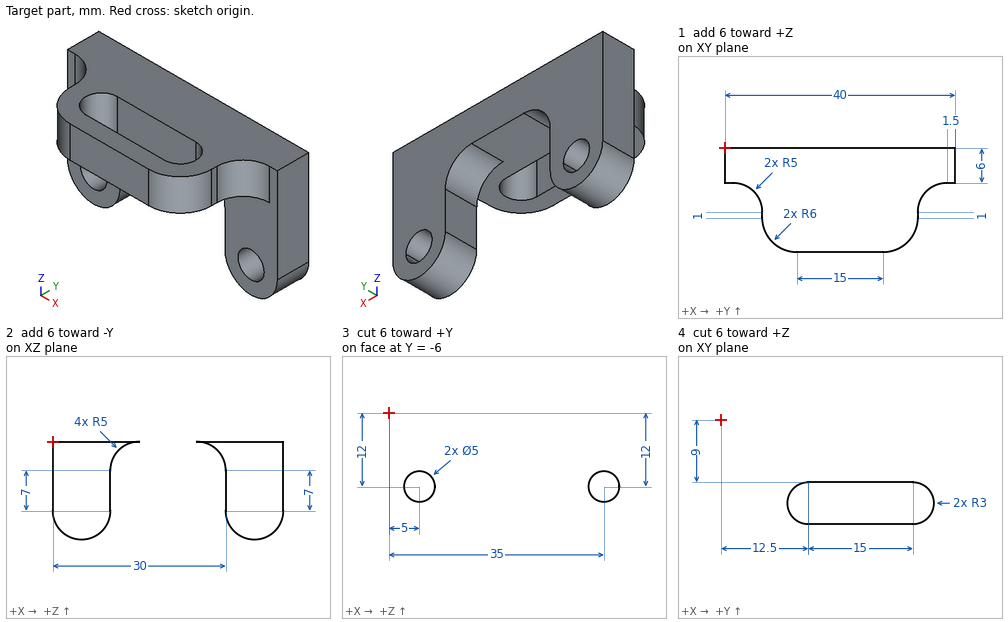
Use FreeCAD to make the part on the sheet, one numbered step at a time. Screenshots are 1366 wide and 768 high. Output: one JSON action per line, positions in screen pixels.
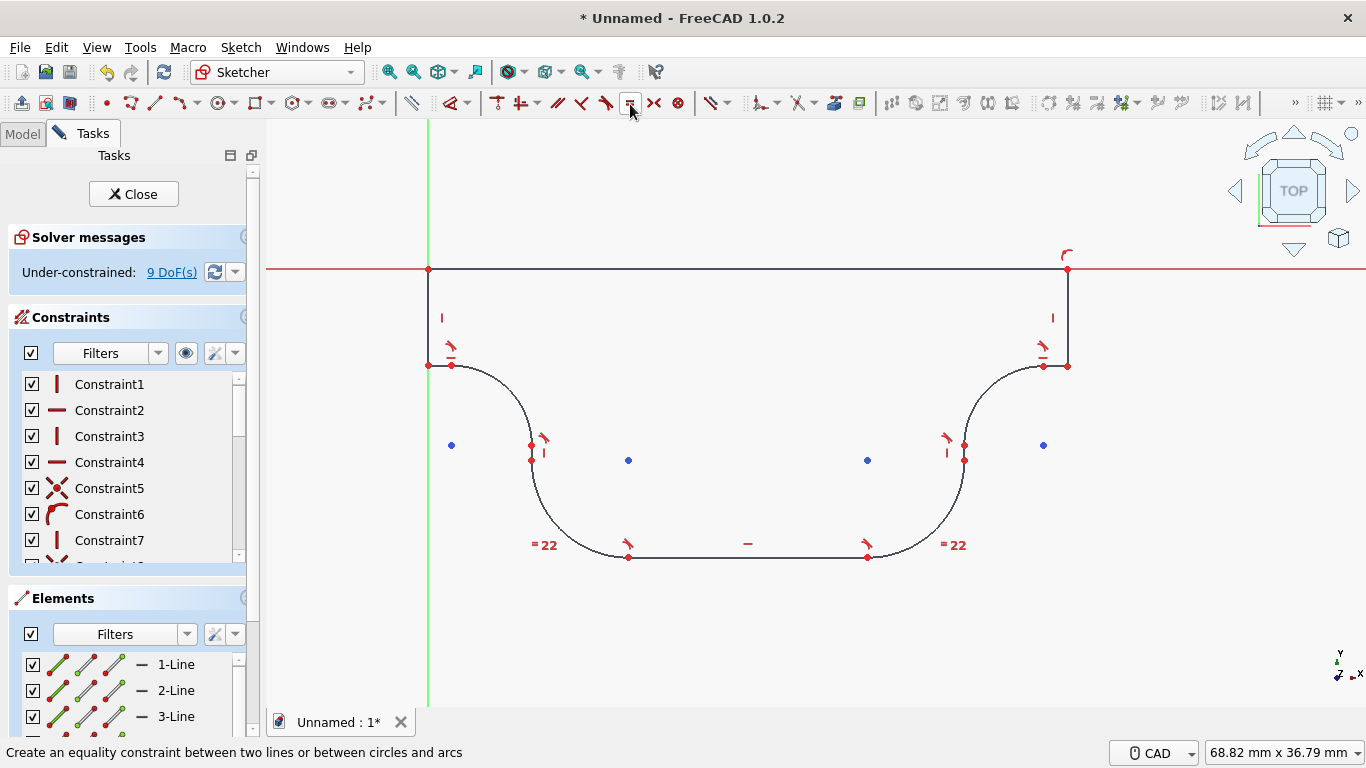
{"action": "left_click", "coordinate": [1008, 375]}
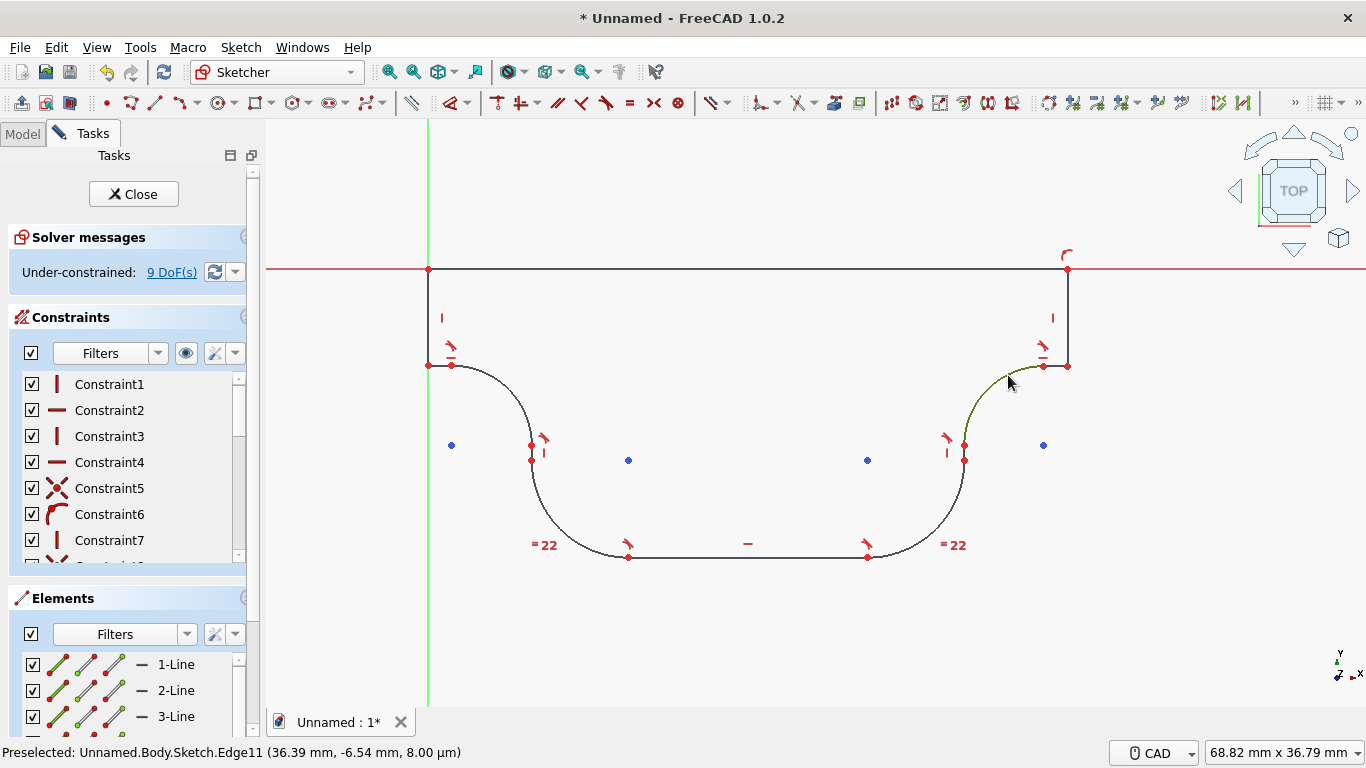
{"action": "left_click", "coordinate": [523, 409]}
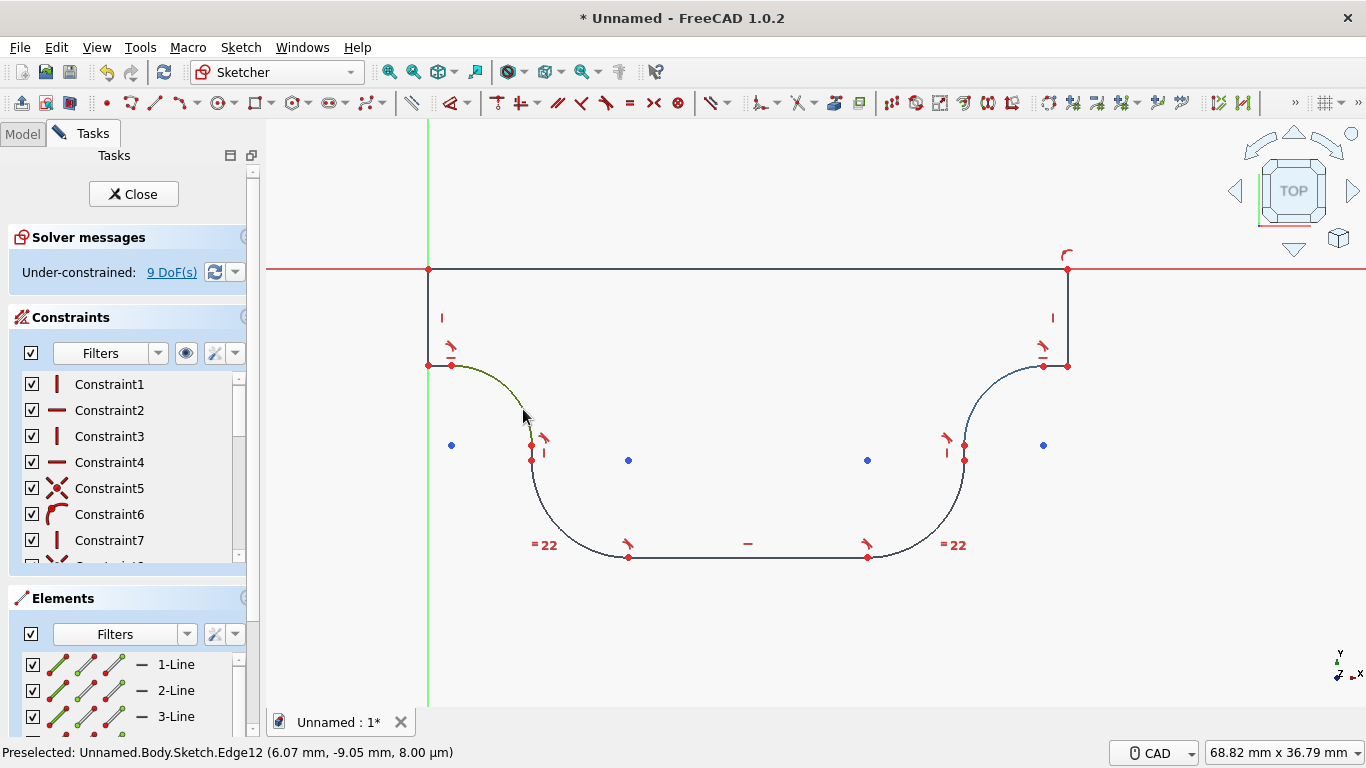
{"action": "key", "text": "e"}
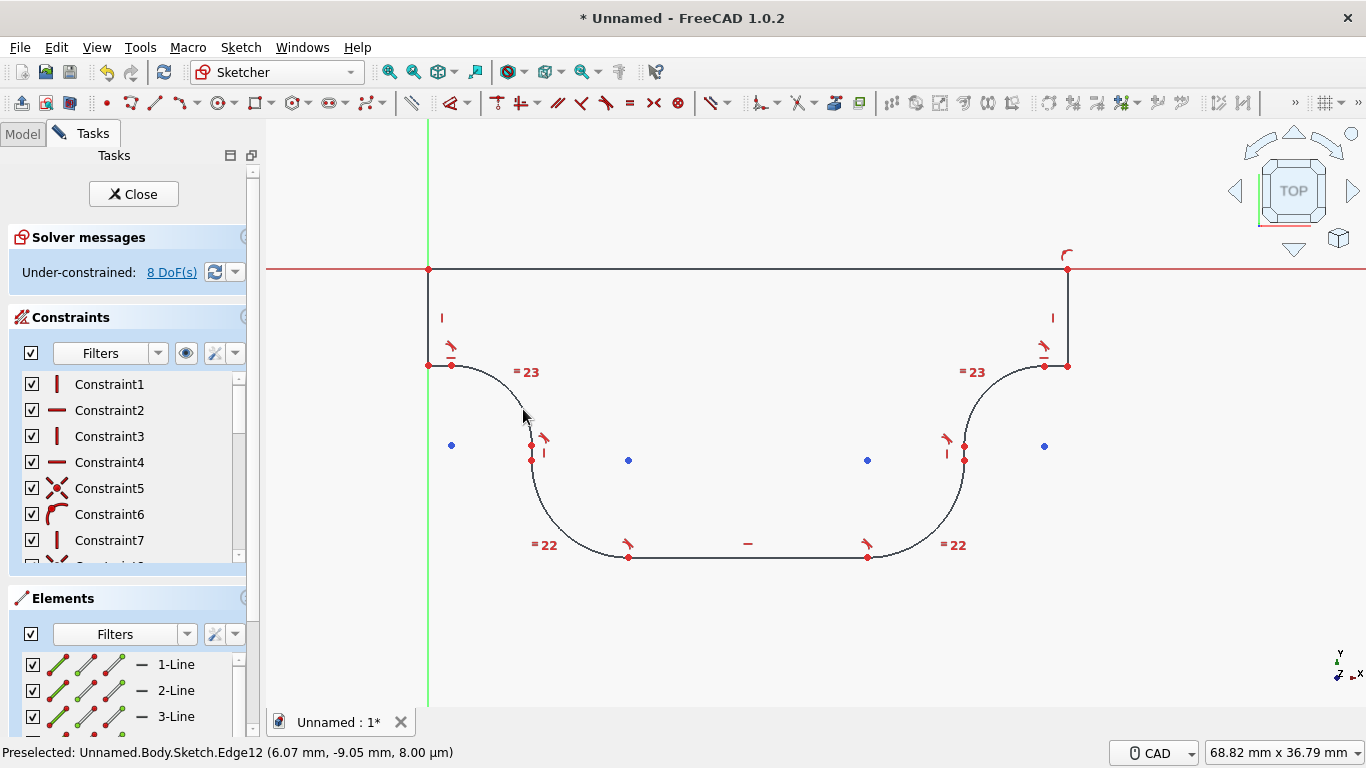
{"action": "key", "text": "d"}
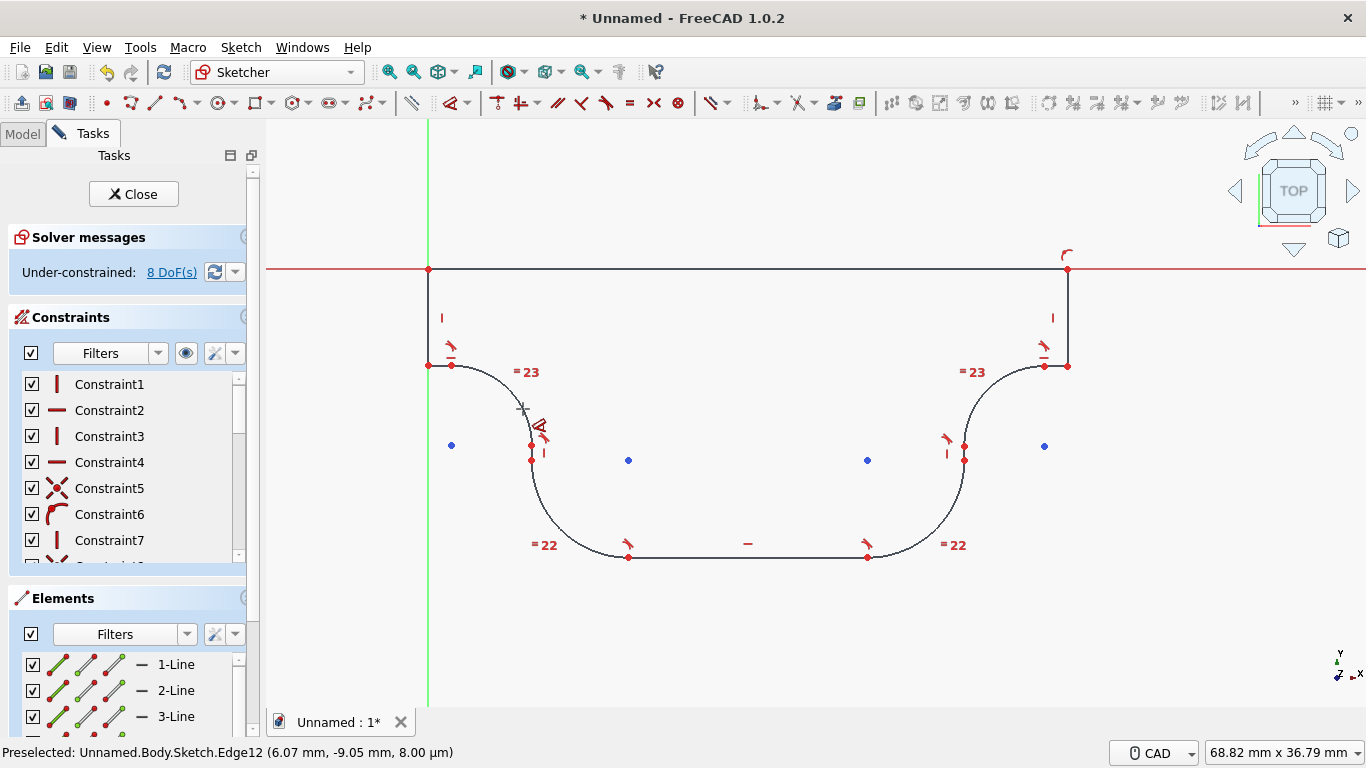
{"action": "left_click", "coordinate": [542, 505]}
{"action": "left_click", "coordinate": [513, 520]}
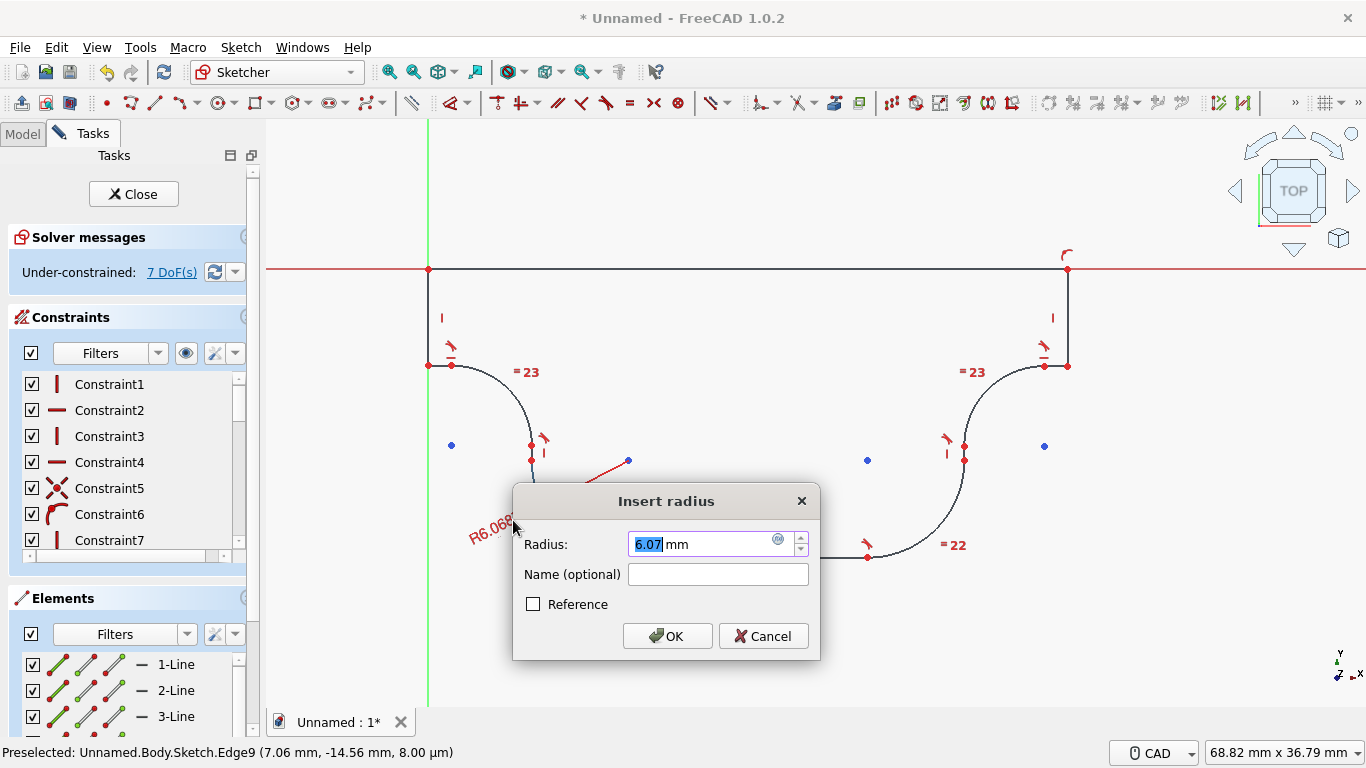
{"action": "type", "text": "6"}
{"action": "key", "text": "Return"}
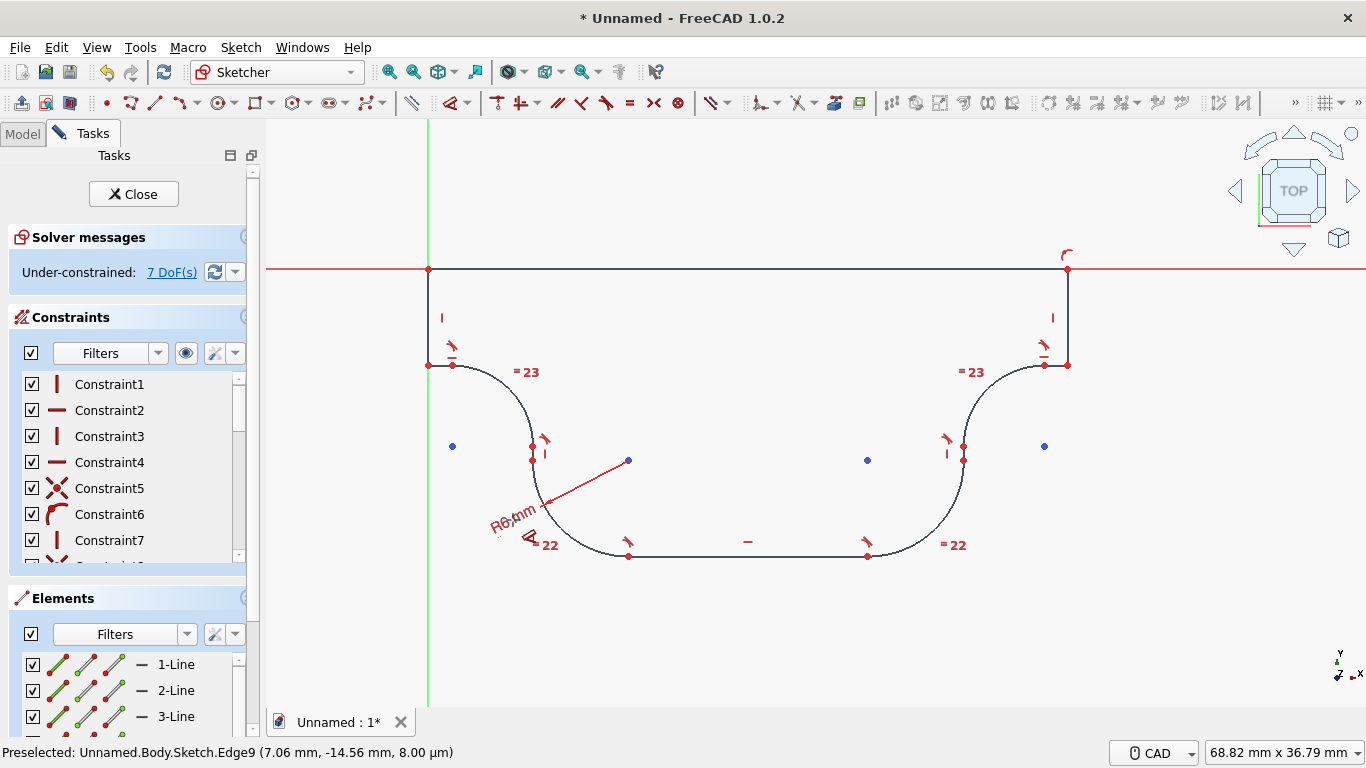
{"action": "left_click", "coordinate": [1008, 374]}
{"action": "left_click", "coordinate": [994, 345]}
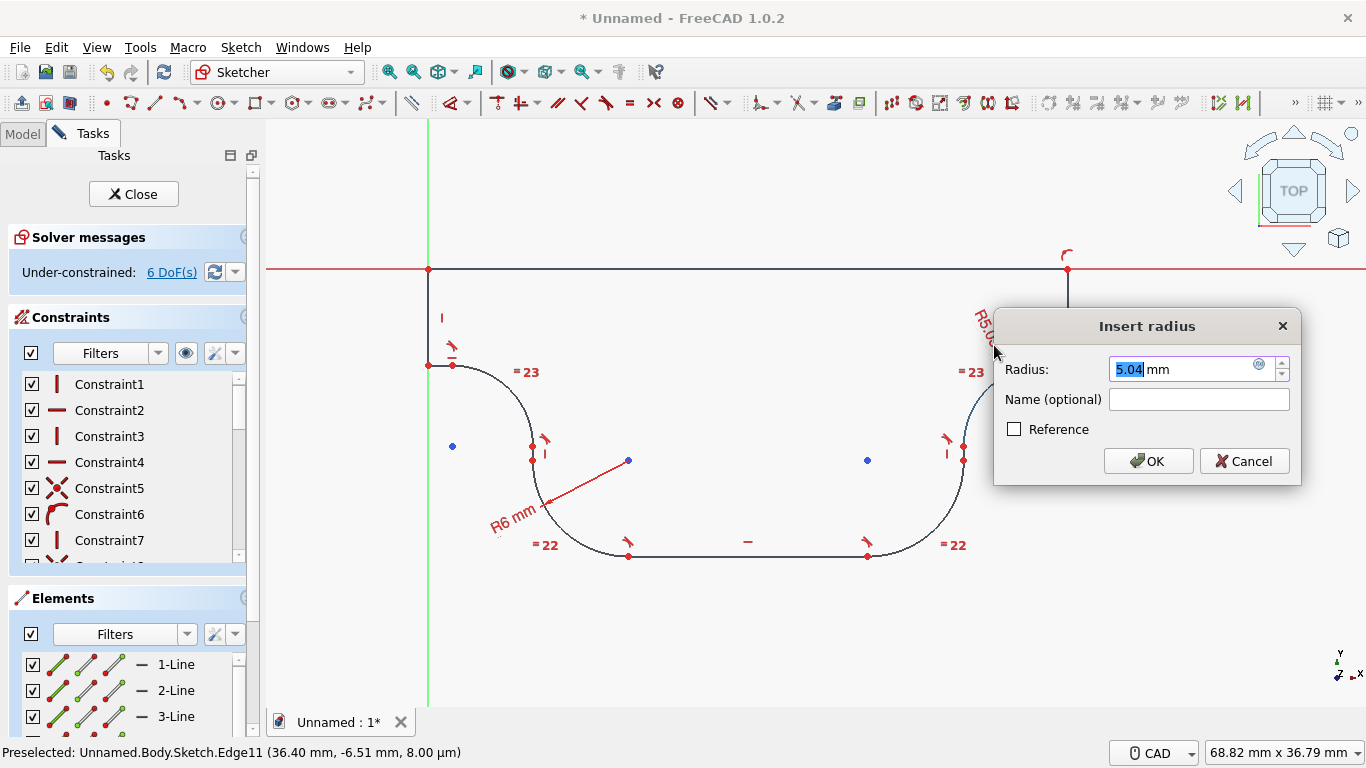
{"action": "type", "text": "5"}
{"action": "key", "text": "Return"}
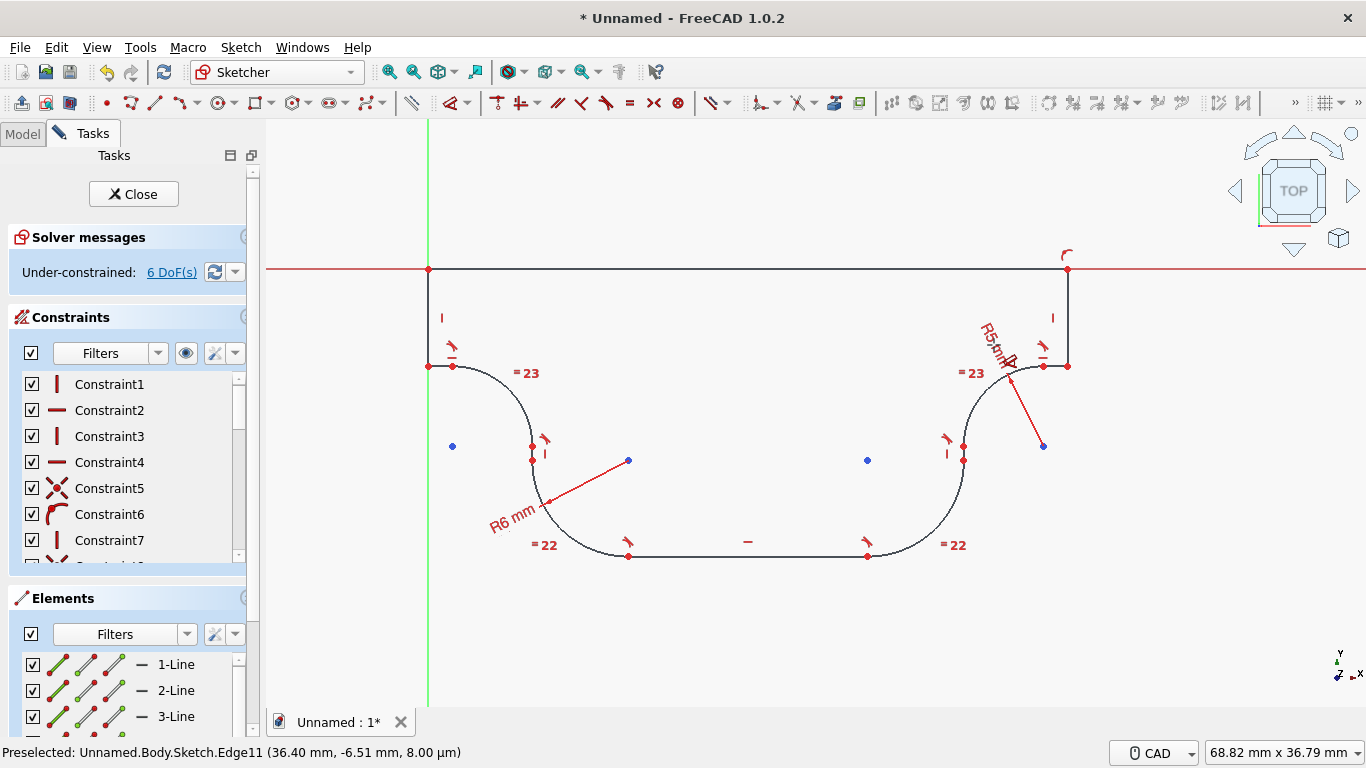
{"action": "scroll", "coordinate": [532, 453], "scroll_direction": "up", "scroll_amount": 5}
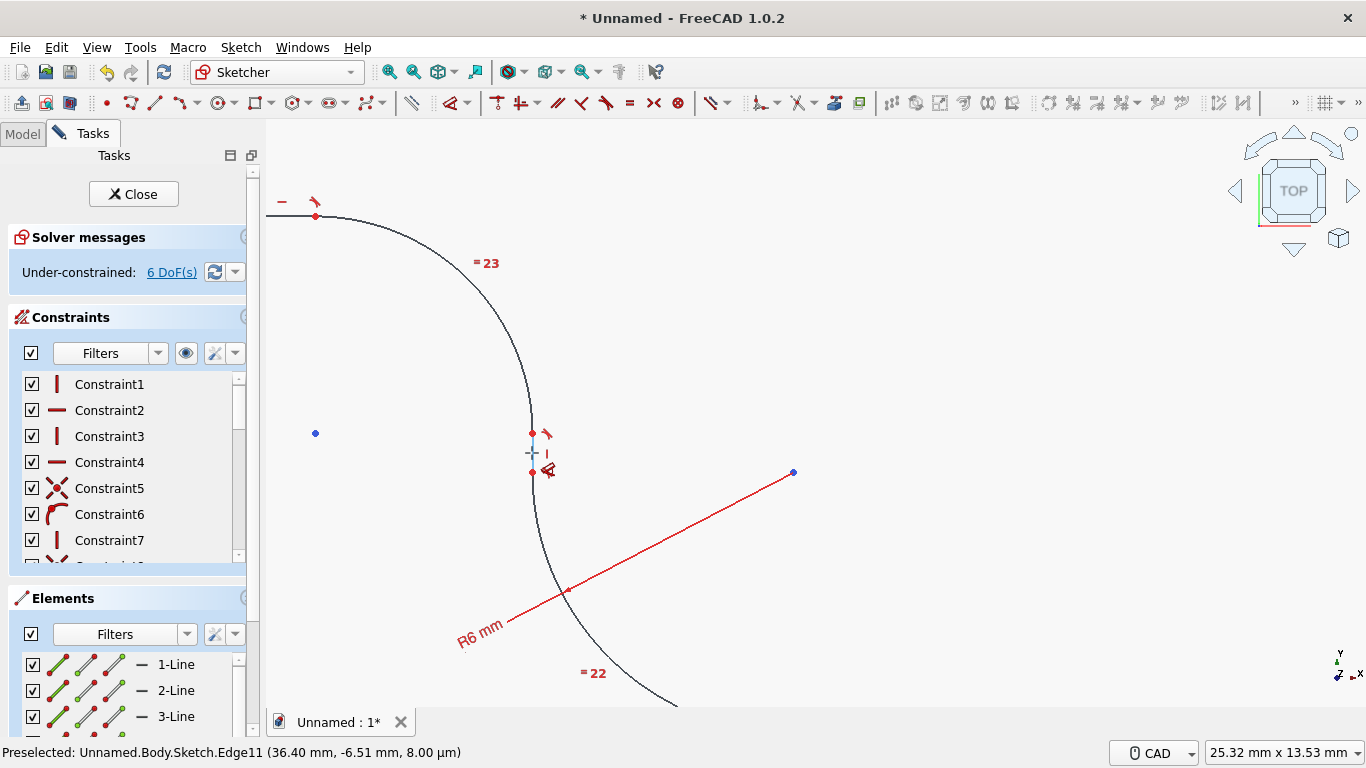
{"action": "left_click", "coordinate": [533, 453]}
{"action": "left_click", "coordinate": [499, 453]}